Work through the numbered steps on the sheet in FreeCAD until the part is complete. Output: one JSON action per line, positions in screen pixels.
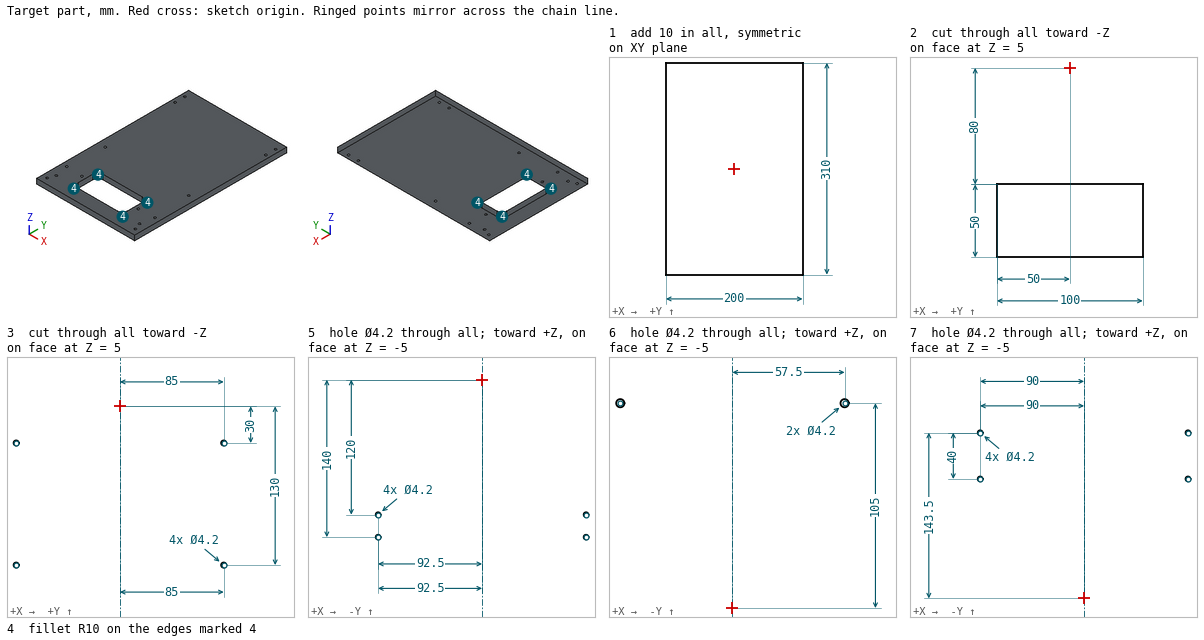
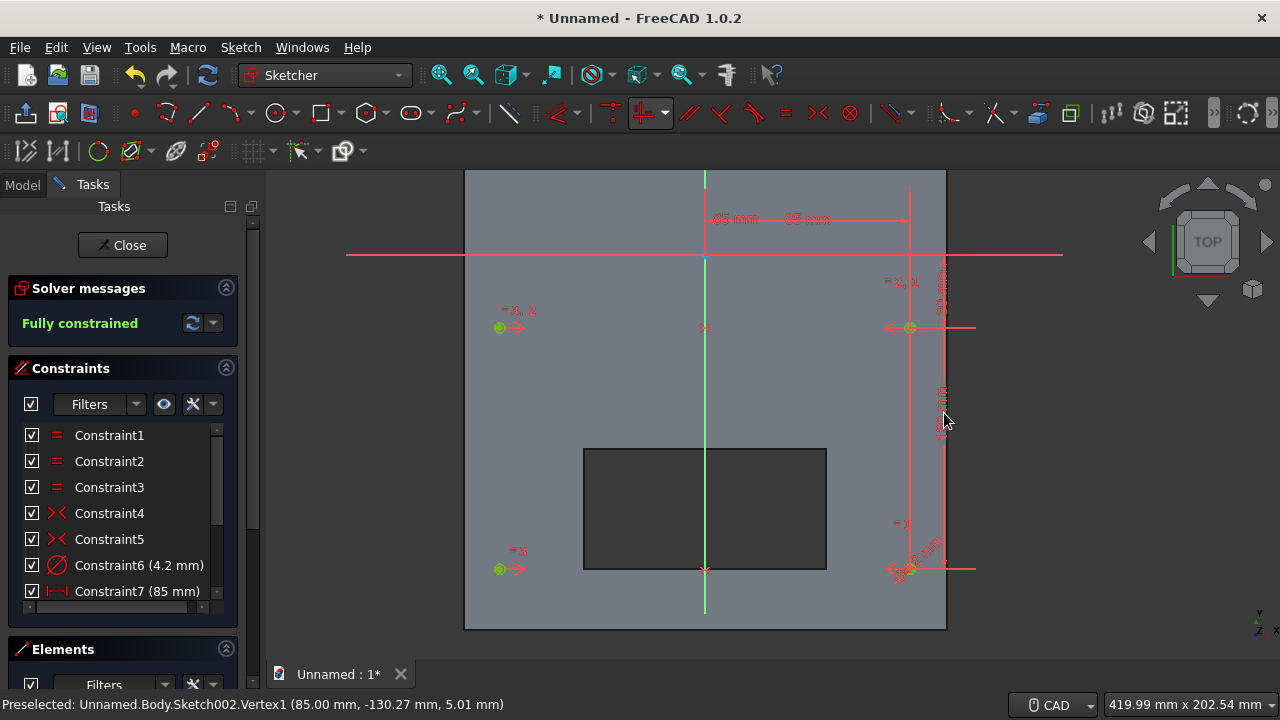
{"action": "left_click", "coordinate": [123, 245]}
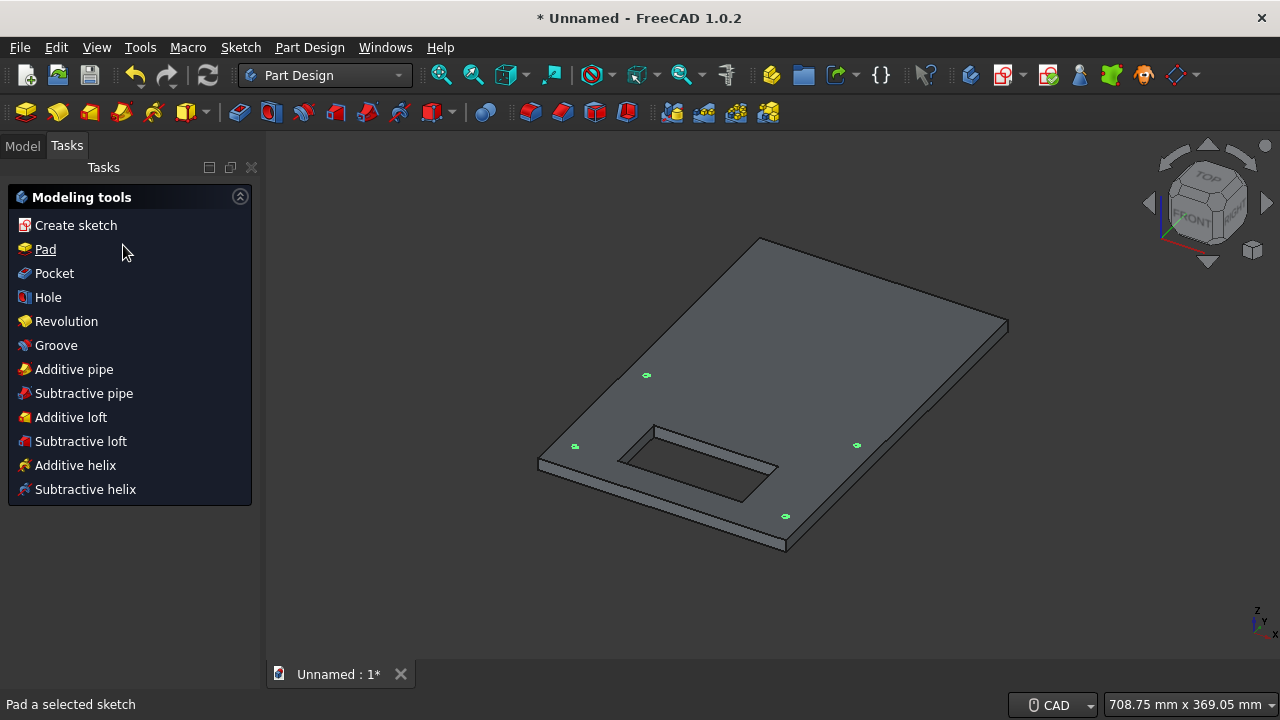
{"action": "left_click", "coordinate": [240, 112]}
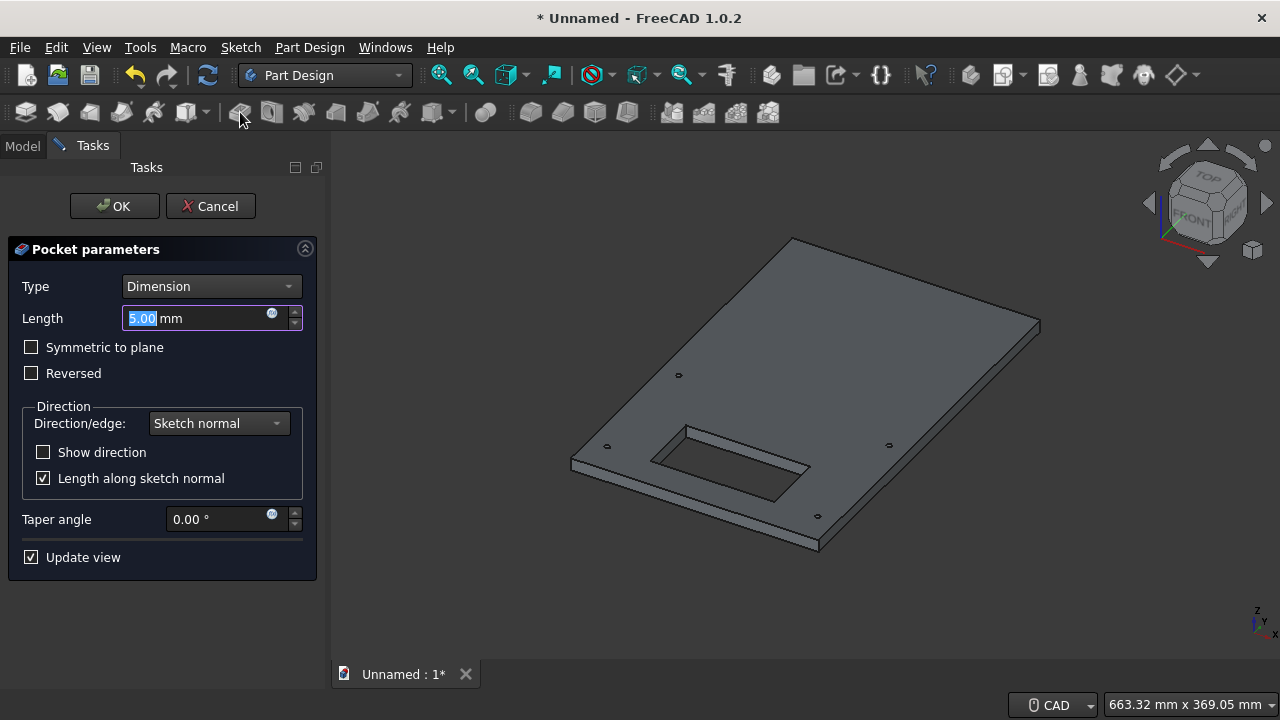
{"action": "left_click", "coordinate": [212, 286]}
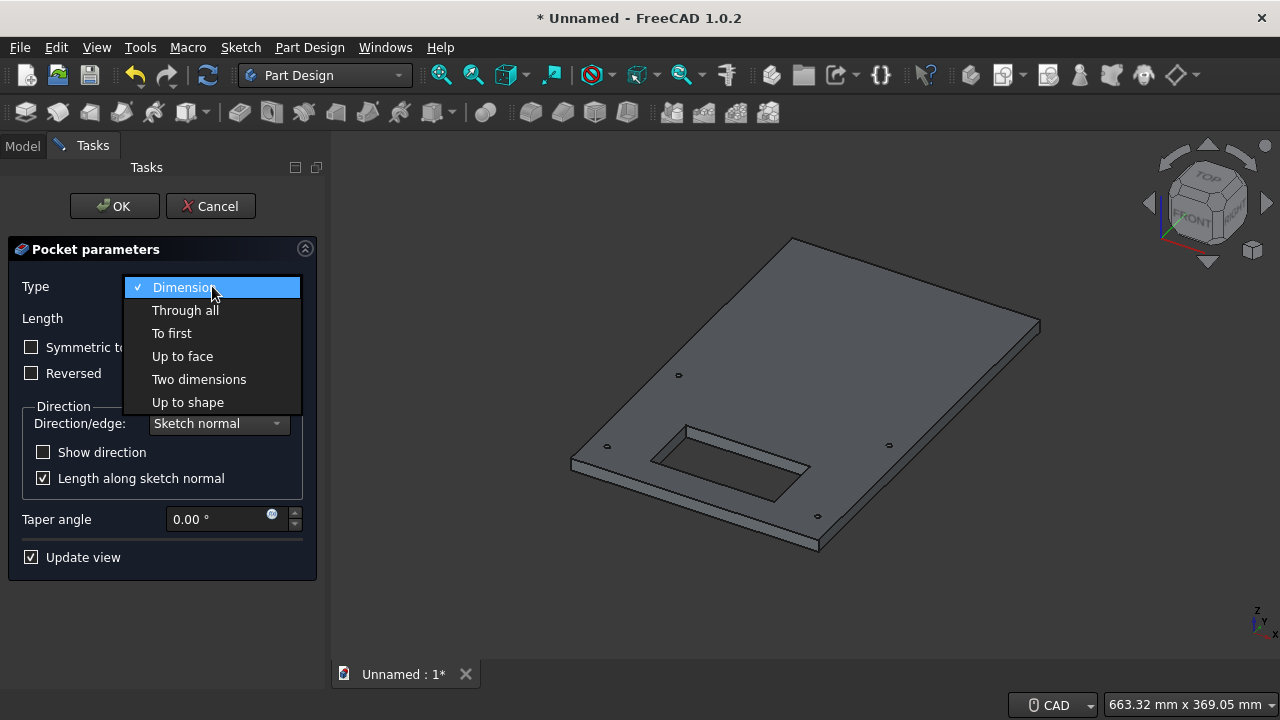
{"action": "left_click", "coordinate": [212, 310]}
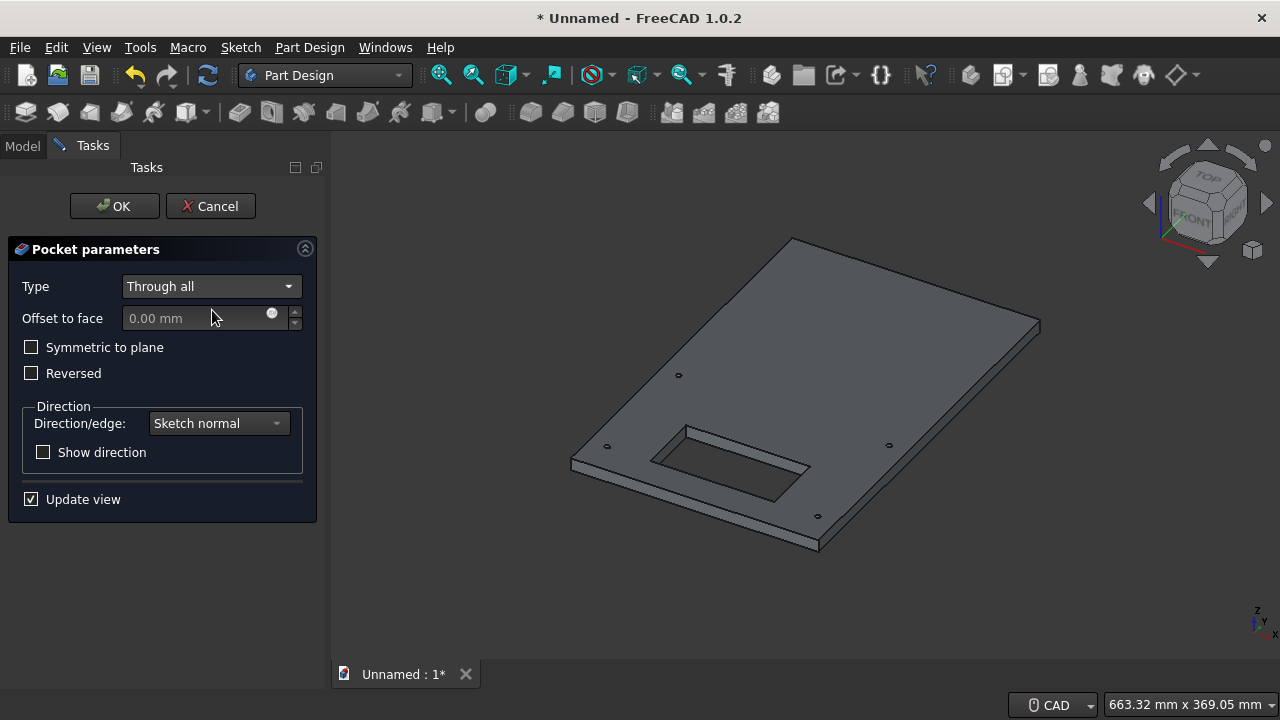
{"action": "left_click", "coordinate": [115, 206]}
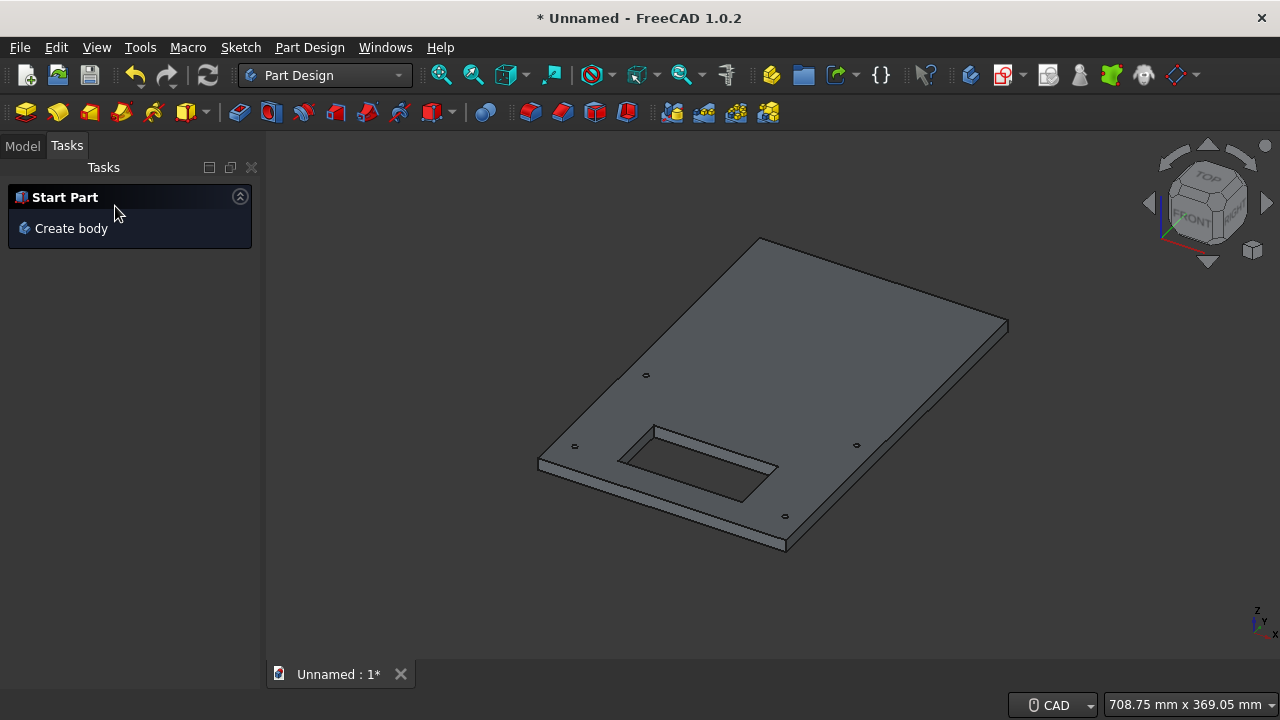
{"action": "scroll", "coordinate": [778, 471], "scroll_direction": "up", "scroll_amount": 6}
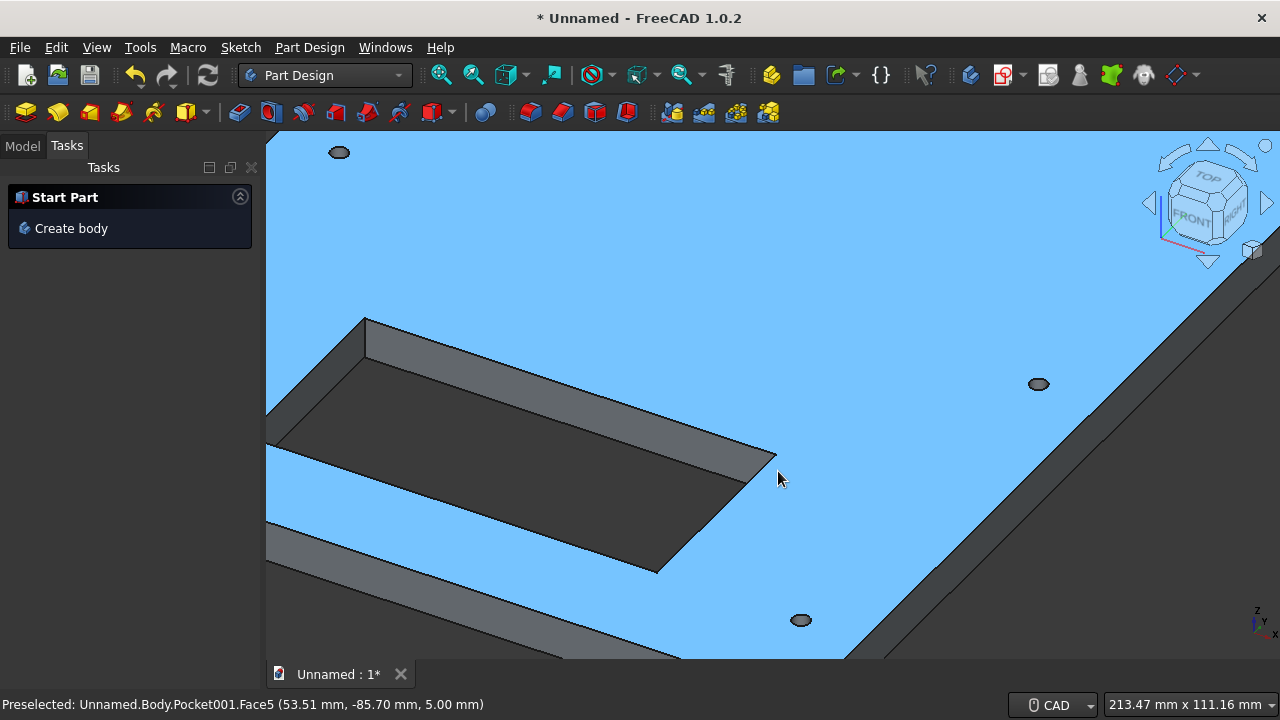
{"action": "left_click", "coordinate": [442, 76]}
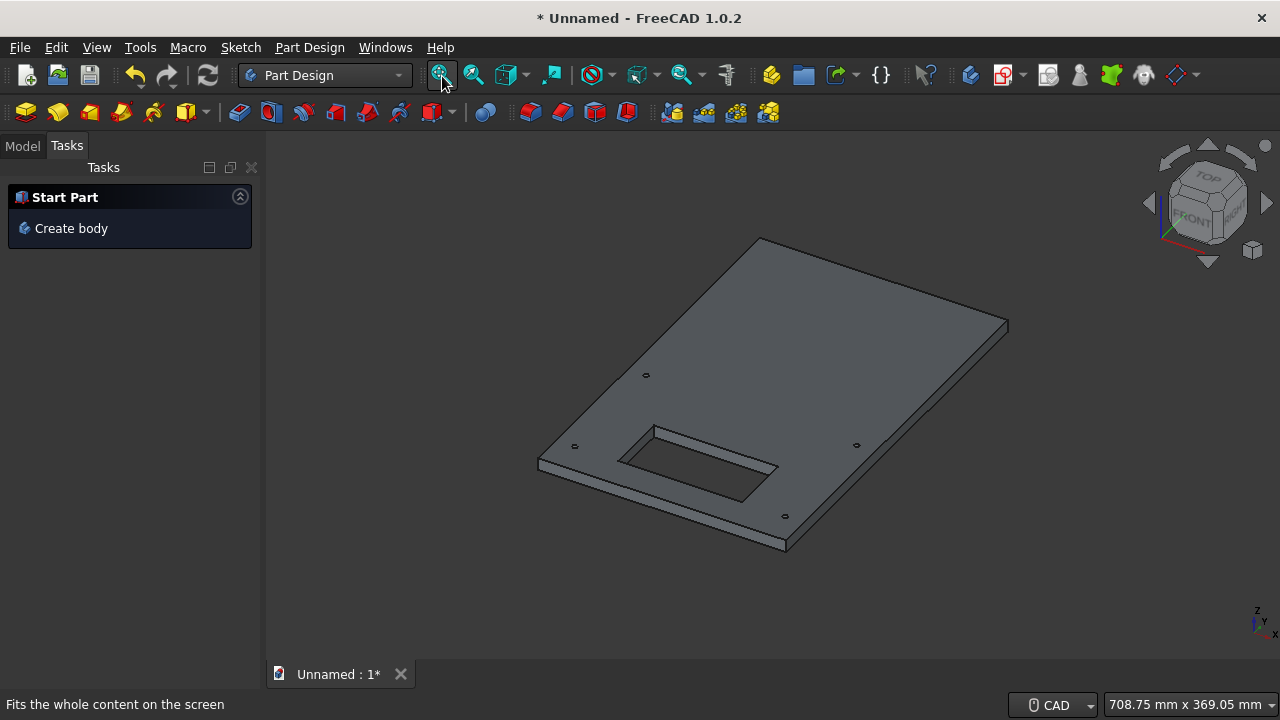
{"action": "key", "text": "0"}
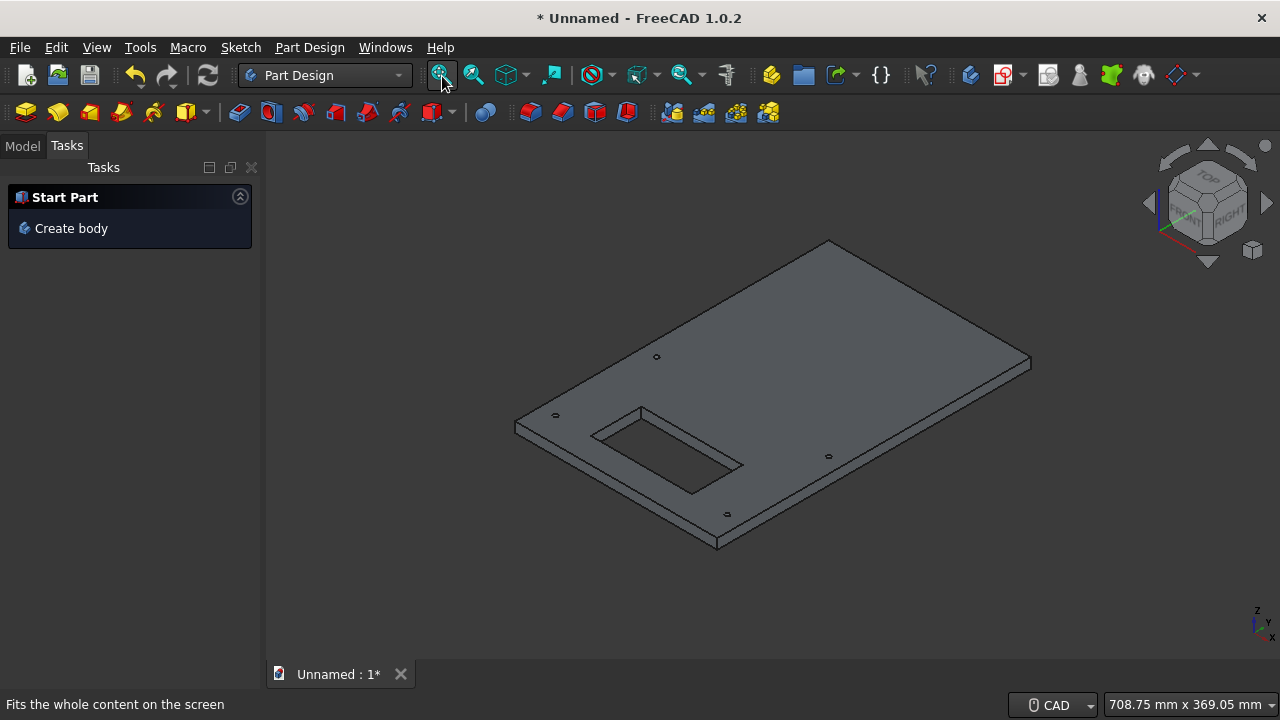
{"action": "scroll", "coordinate": [743, 470], "scroll_direction": "up", "scroll_amount": 6}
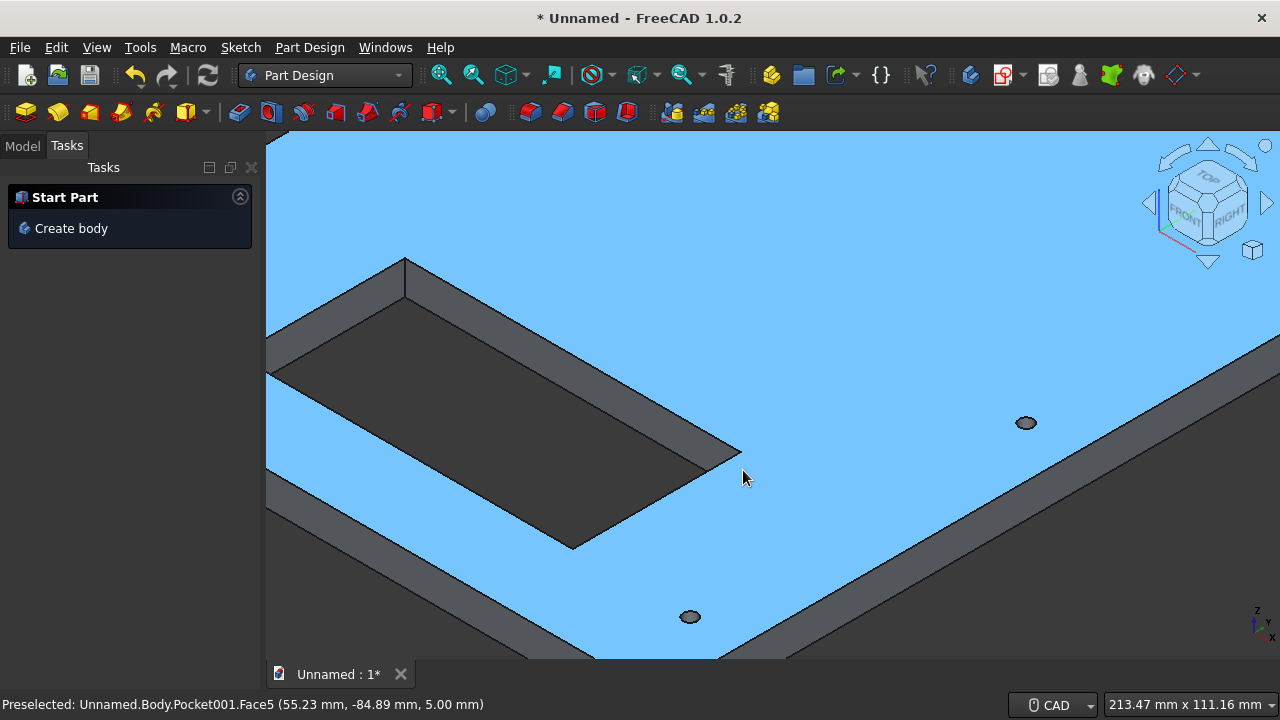
{"action": "left_click", "coordinate": [442, 76]}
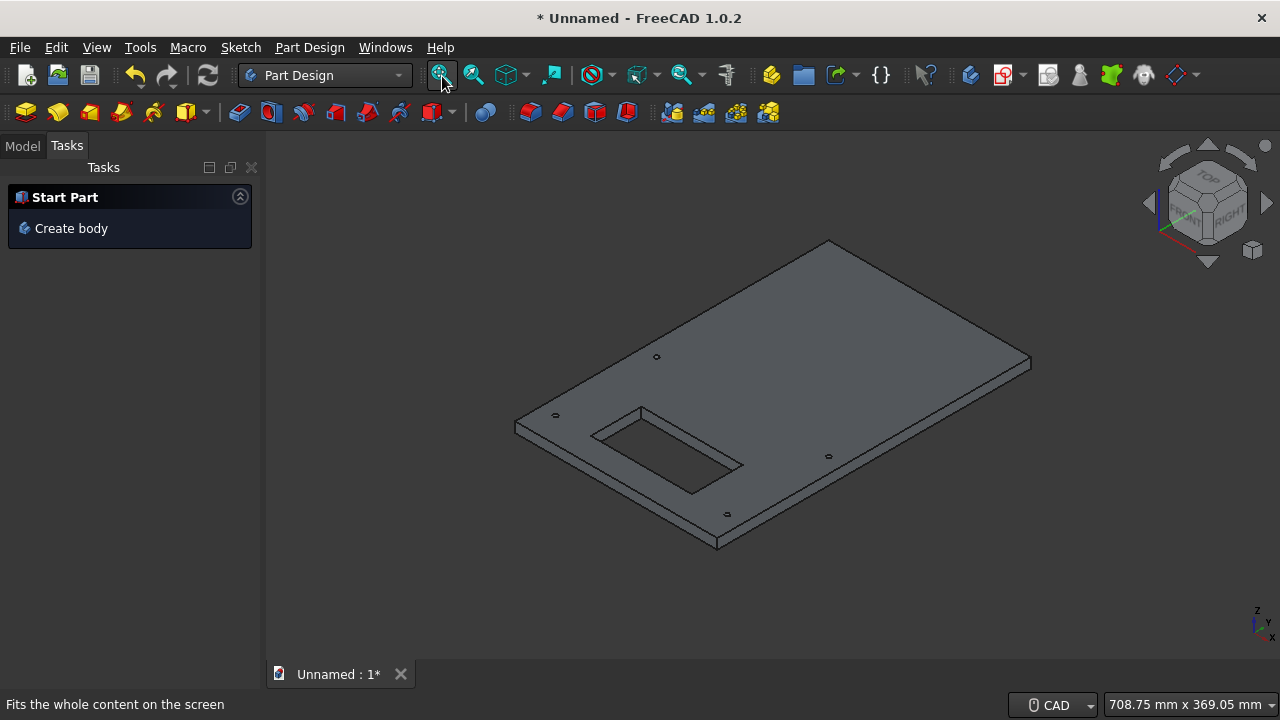
{"action": "key", "text": "2"}